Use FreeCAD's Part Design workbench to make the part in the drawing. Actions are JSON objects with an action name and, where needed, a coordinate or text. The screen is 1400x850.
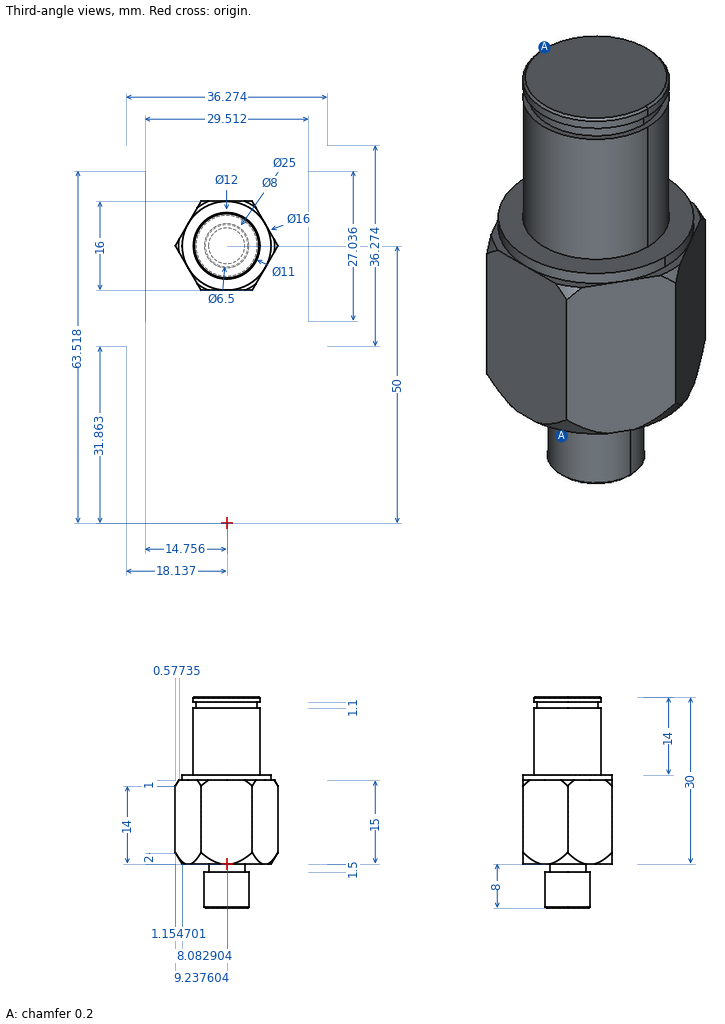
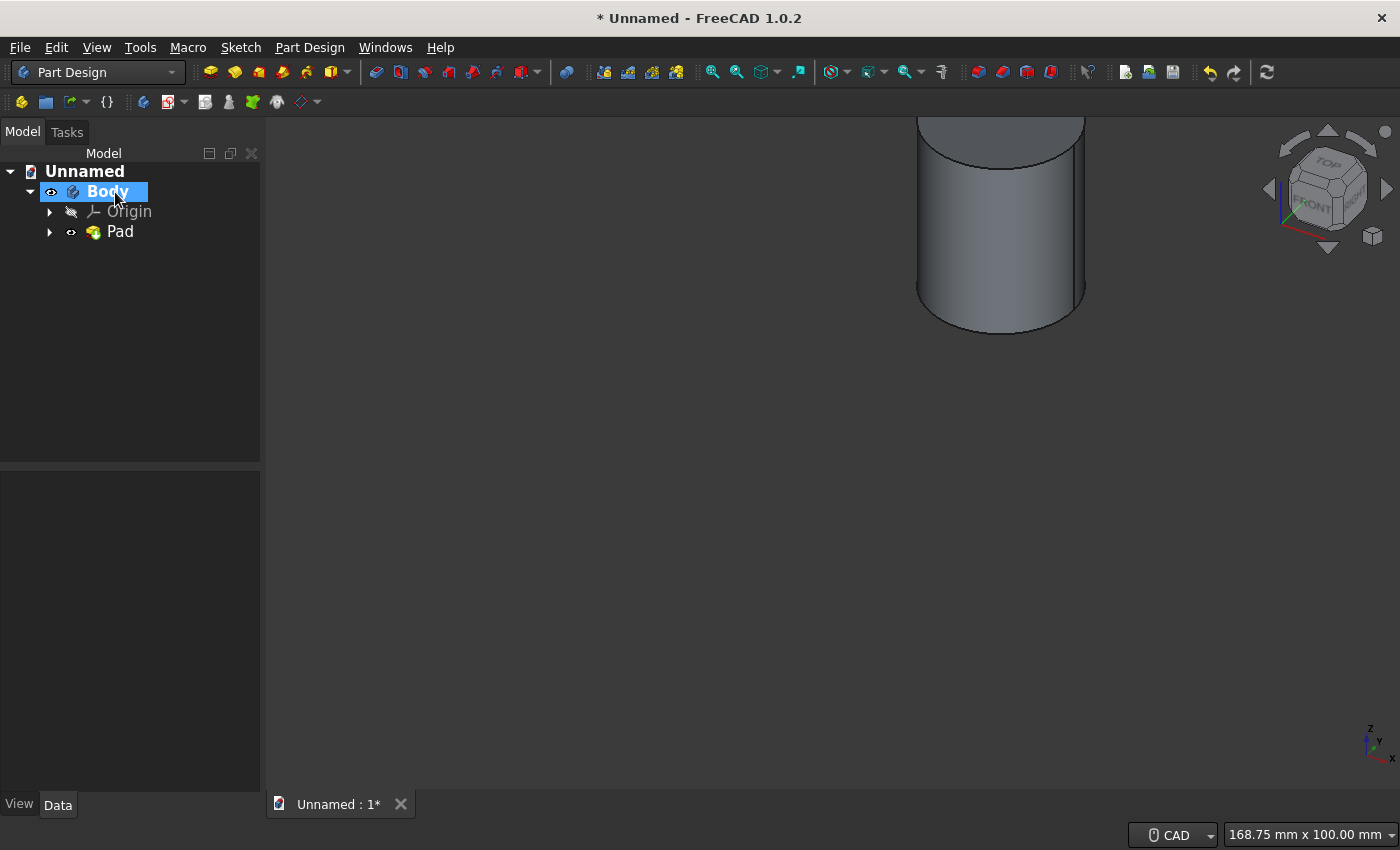
{"action": "left_click", "coordinate": [714, 72]}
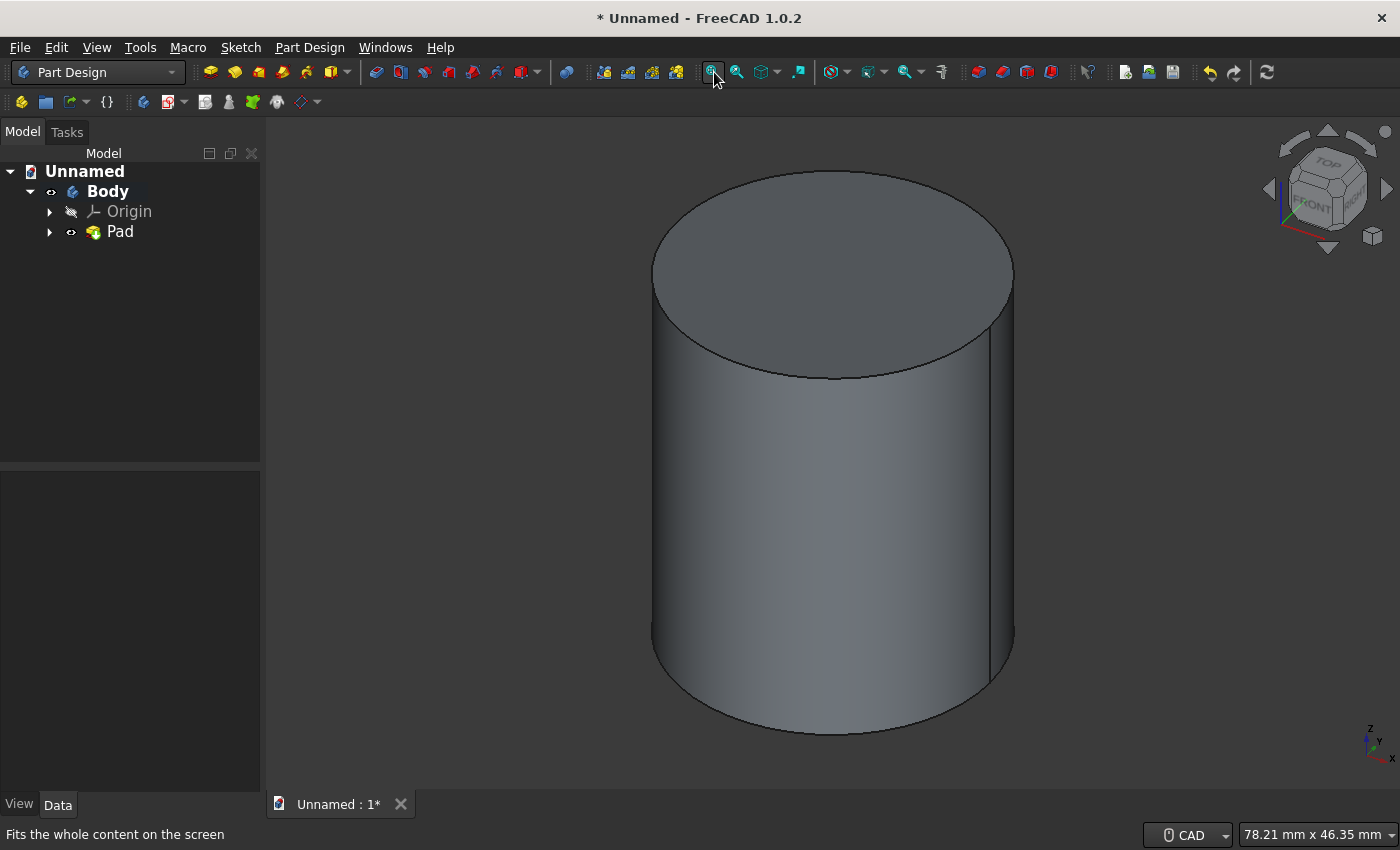
{"action": "key", "text": "5"}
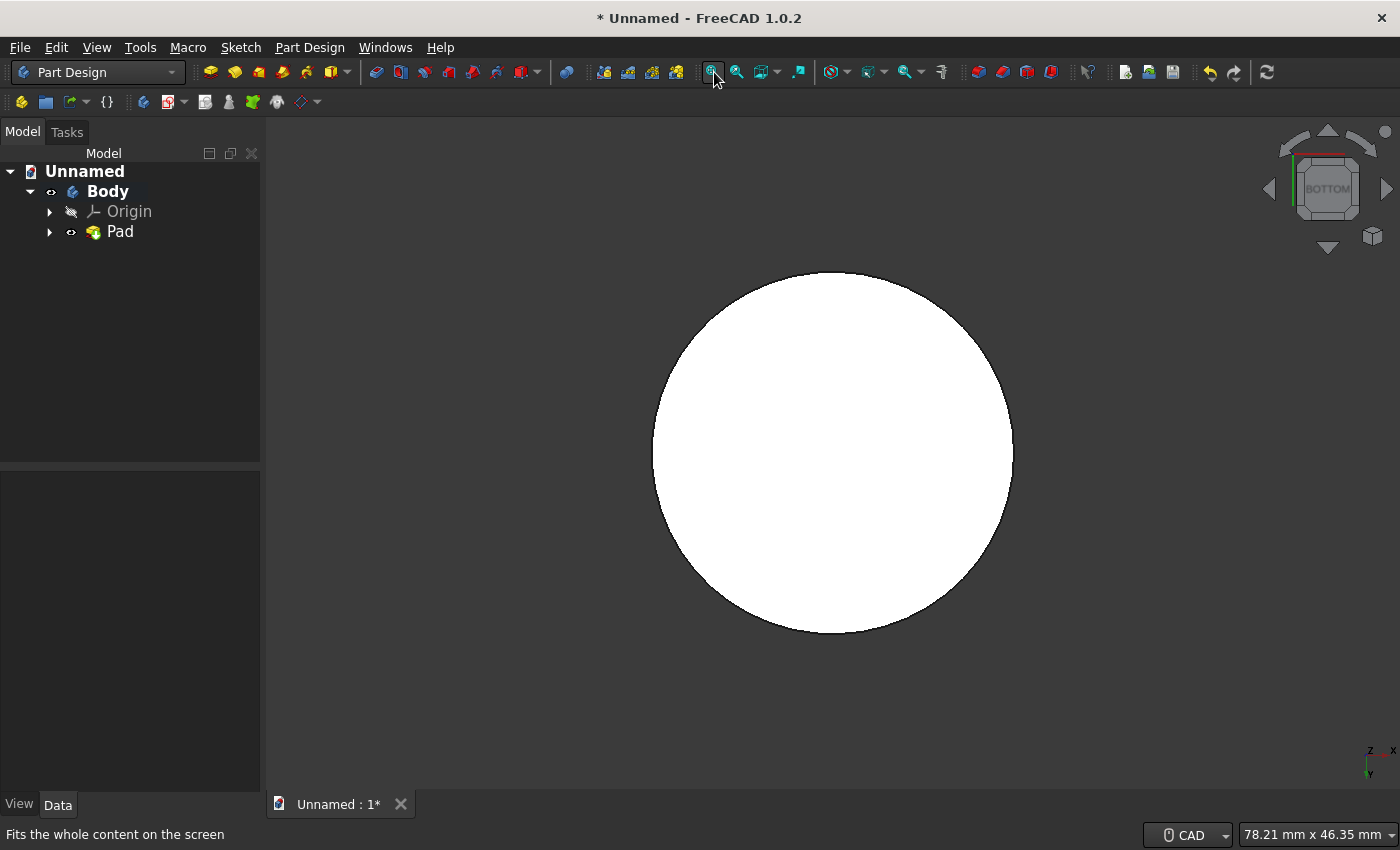
{"action": "left_click", "coordinate": [833, 452]}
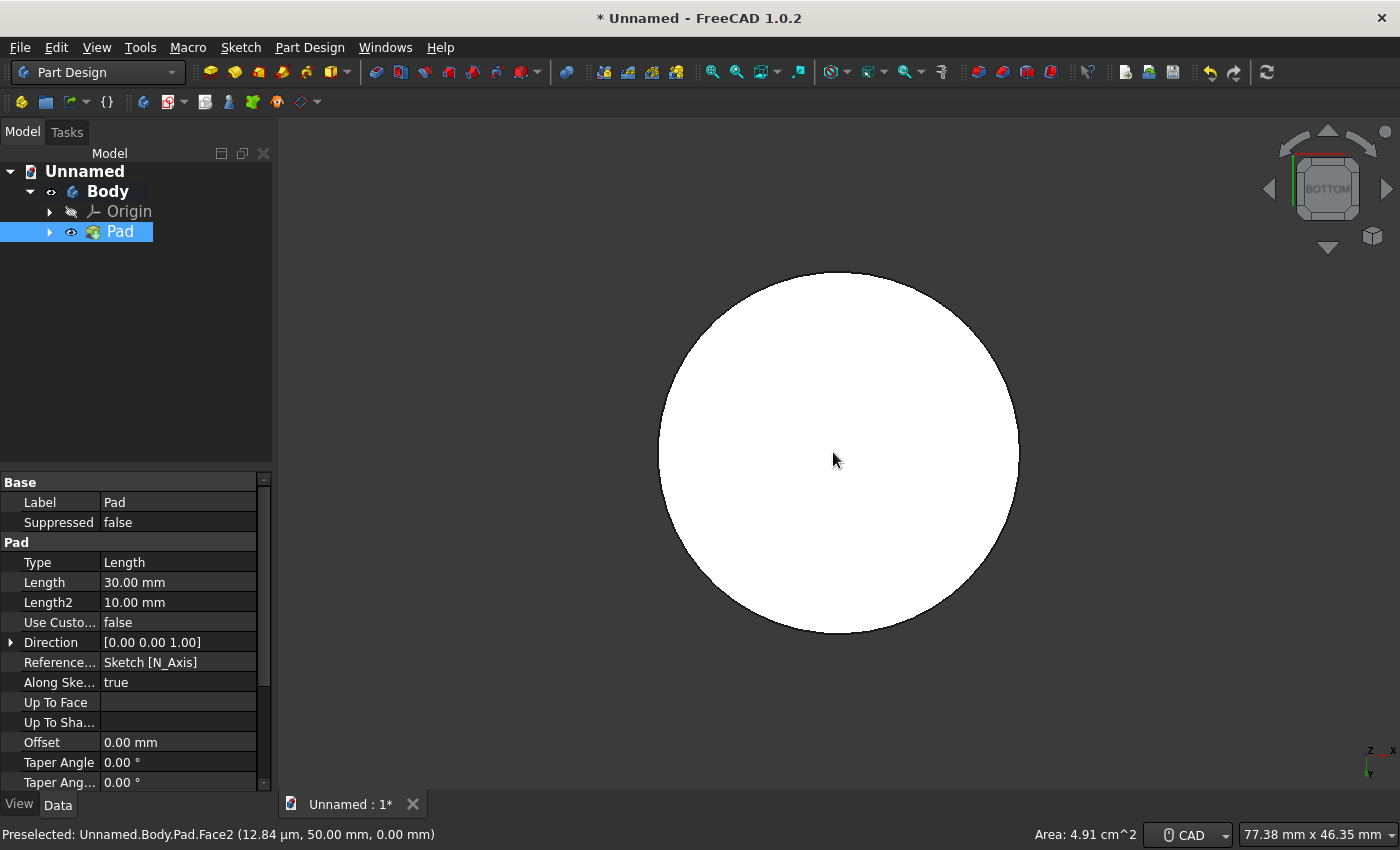
{"action": "left_click", "coordinate": [168, 102]}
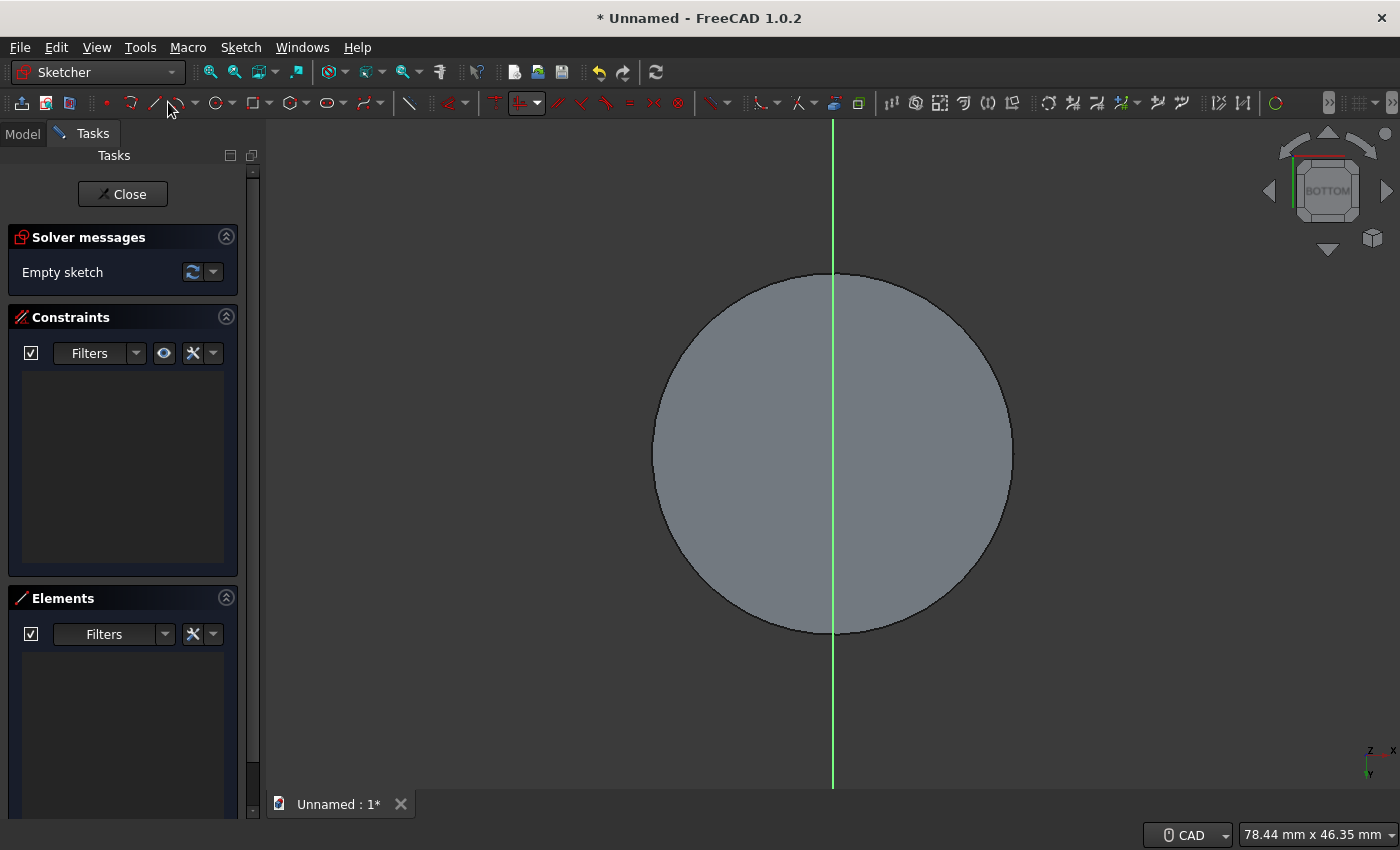
{"action": "scroll", "coordinate": [709, 642], "scroll_direction": "down", "scroll_amount": 4}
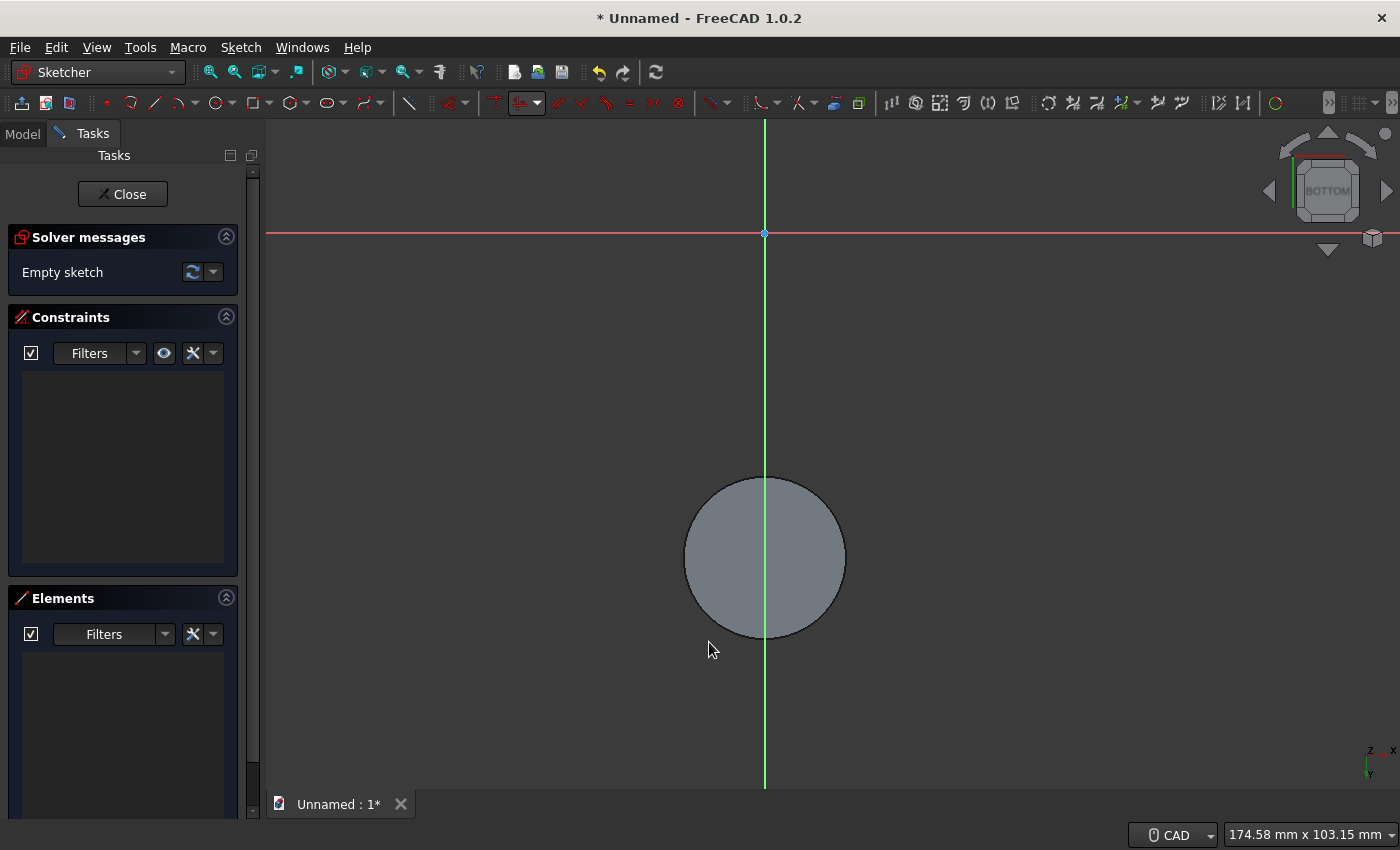
{"action": "left_click", "coordinate": [254, 104]}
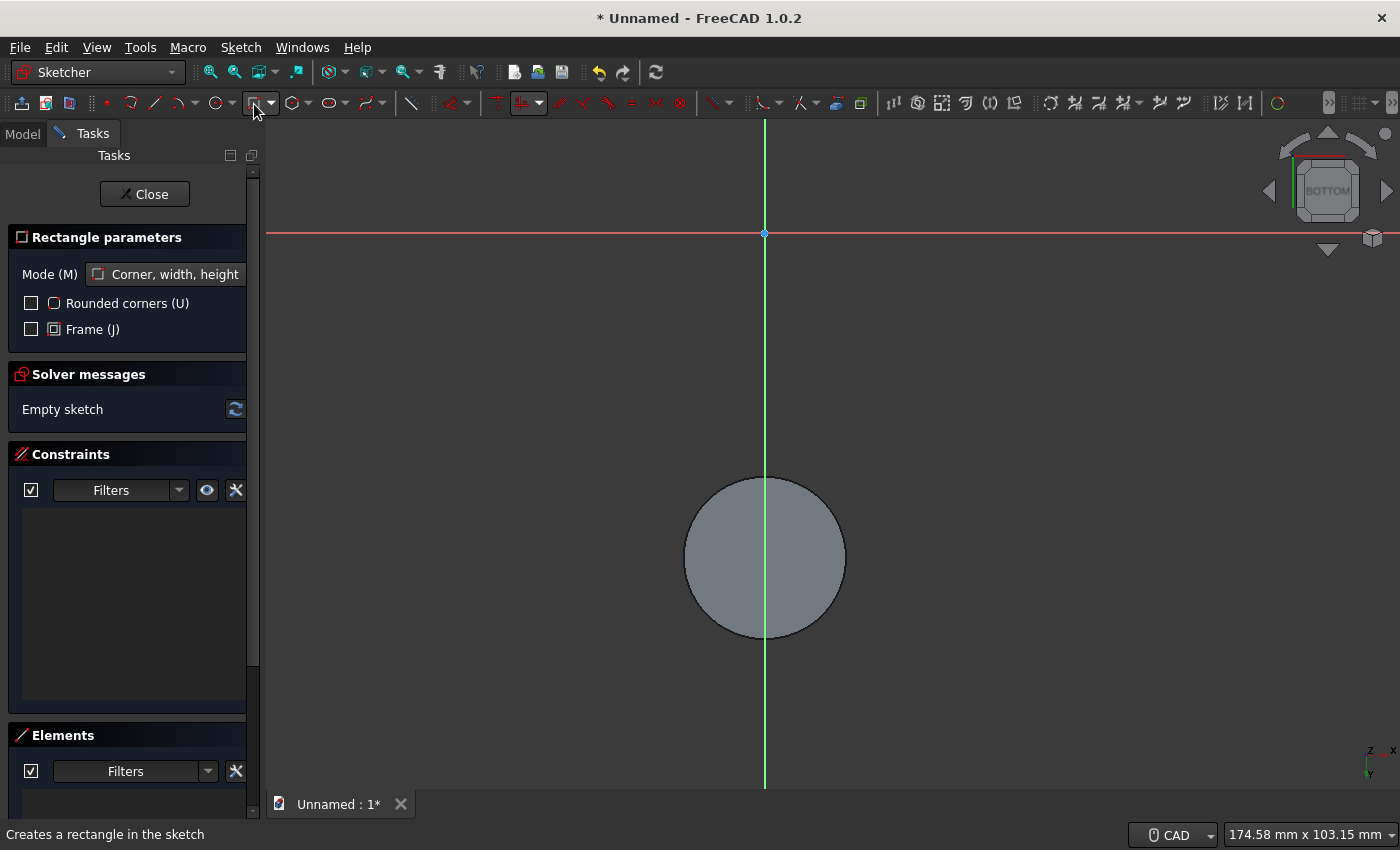
{"action": "left_click", "coordinate": [647, 440]}
{"action": "mouse_move", "coordinate": [883, 676]}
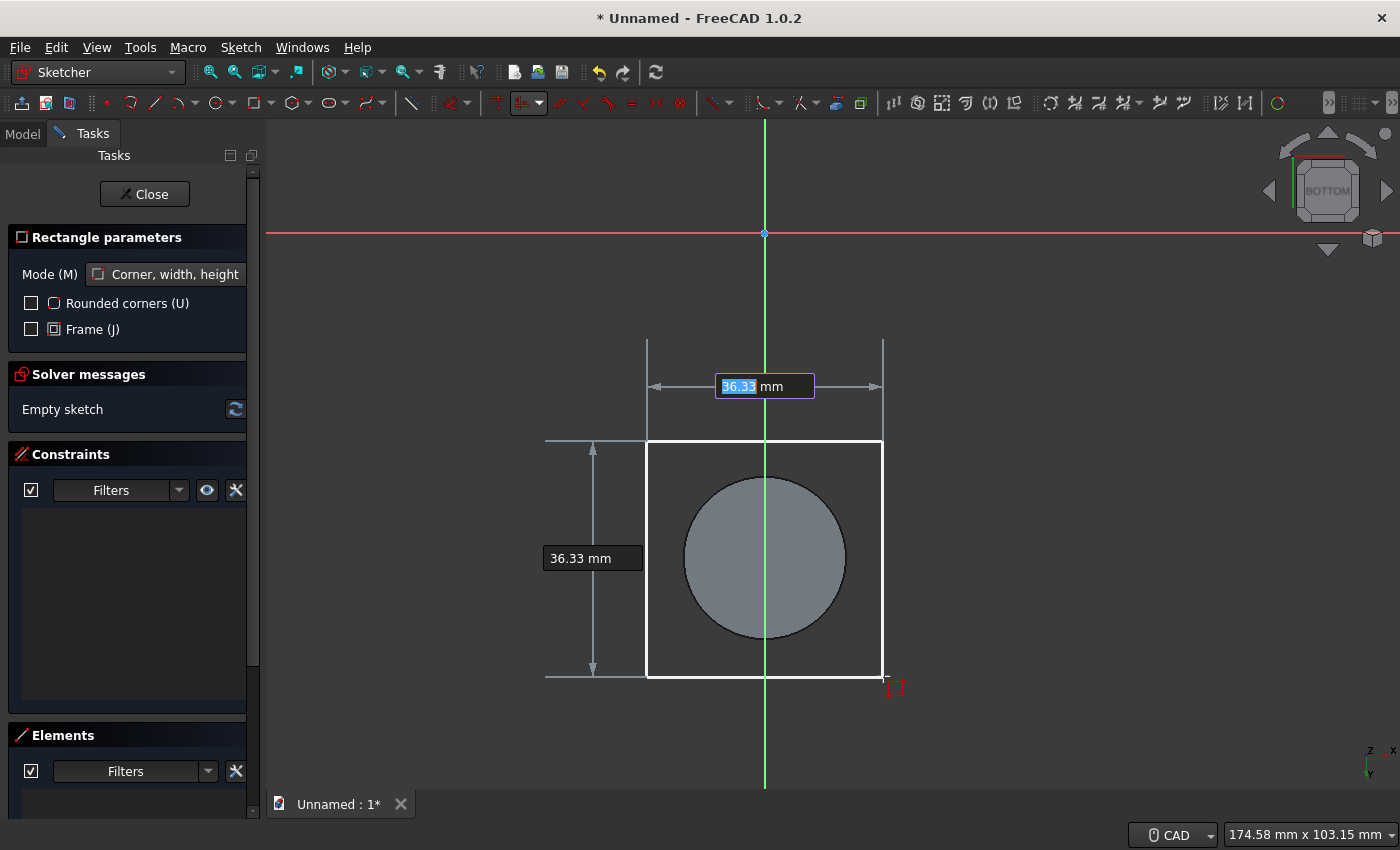
{"action": "type", "text": "36.274"}
{"action": "key", "text": "Tab"}
{"action": "type", "text": "36.274"}
{"action": "key", "text": "Return"}